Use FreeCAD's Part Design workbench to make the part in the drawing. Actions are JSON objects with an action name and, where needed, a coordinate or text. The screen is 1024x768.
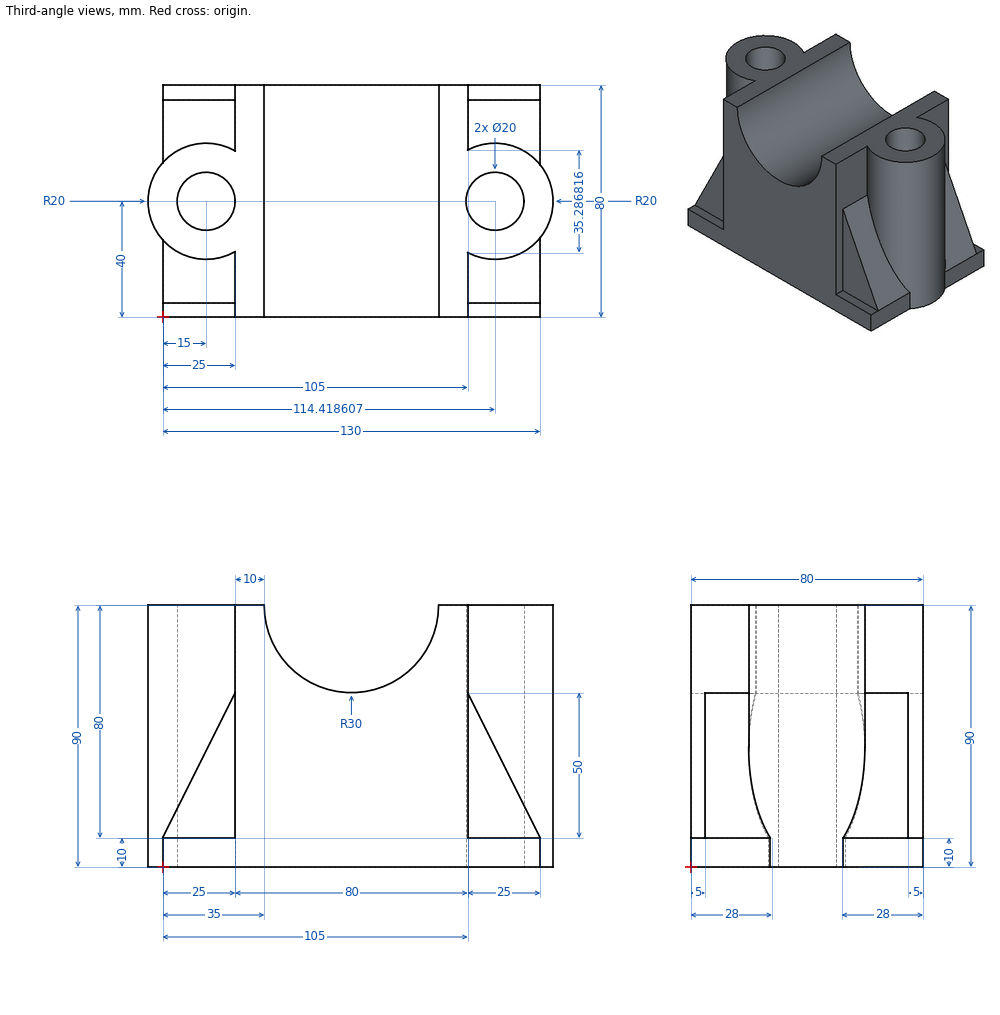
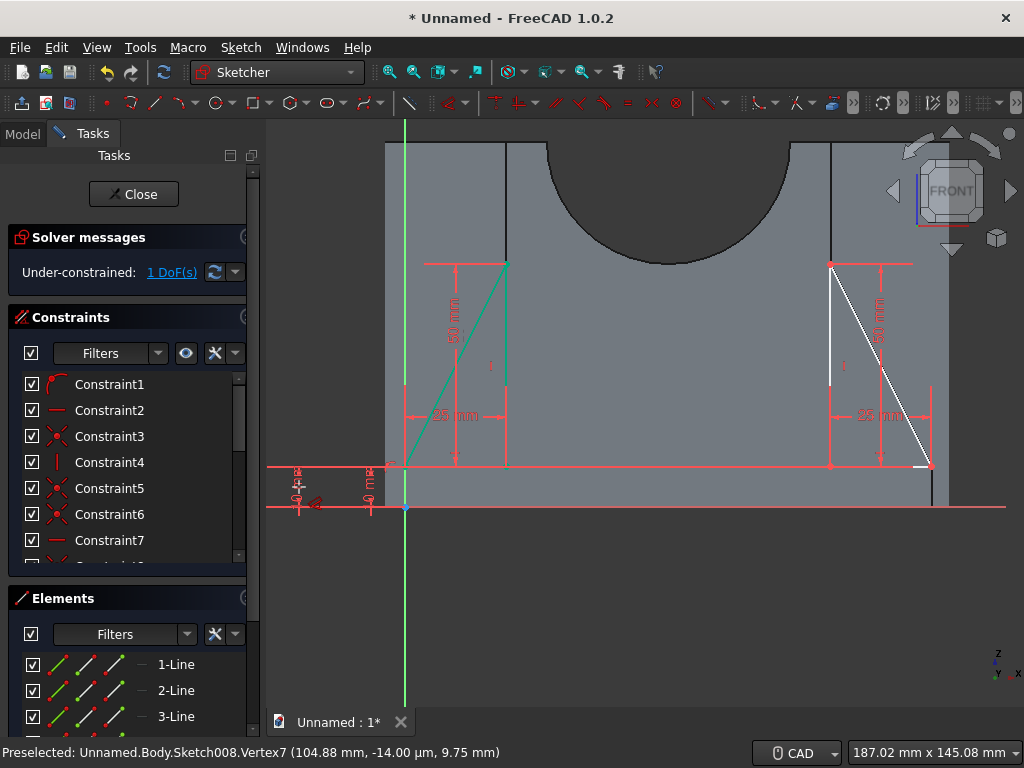
{"action": "left_click", "coordinate": [830, 467]}
{"action": "left_click", "coordinate": [618, 541]}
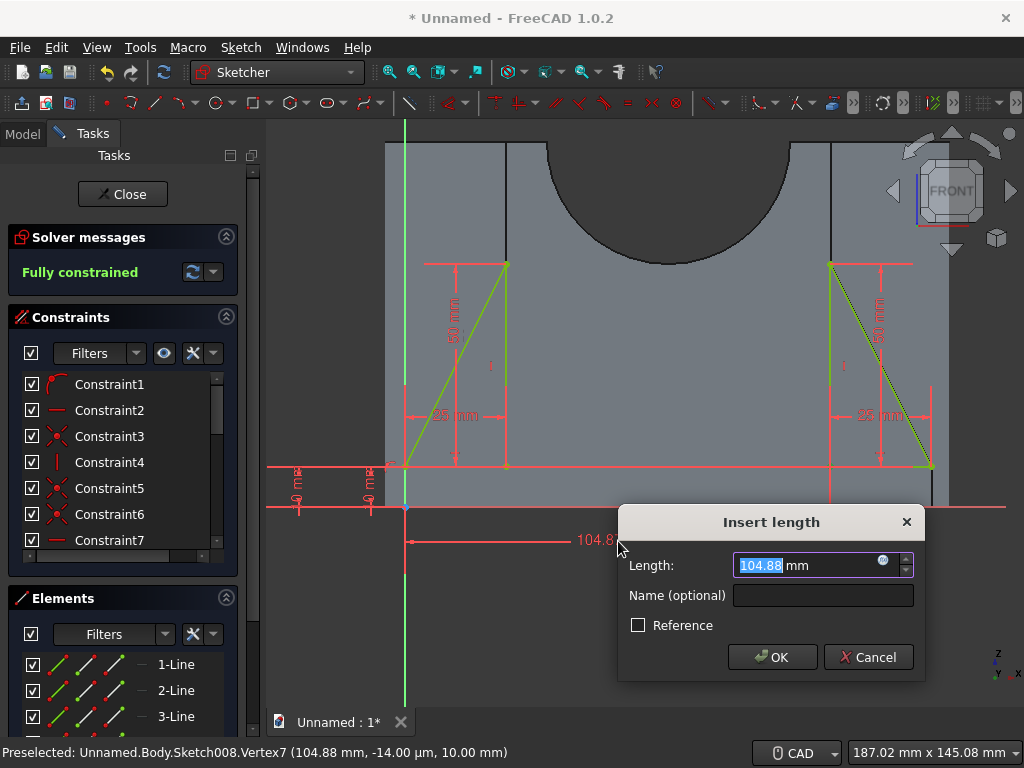
{"action": "type", "text": "105"}
{"action": "key", "text": "Return"}
{"action": "key", "text": "Escape"}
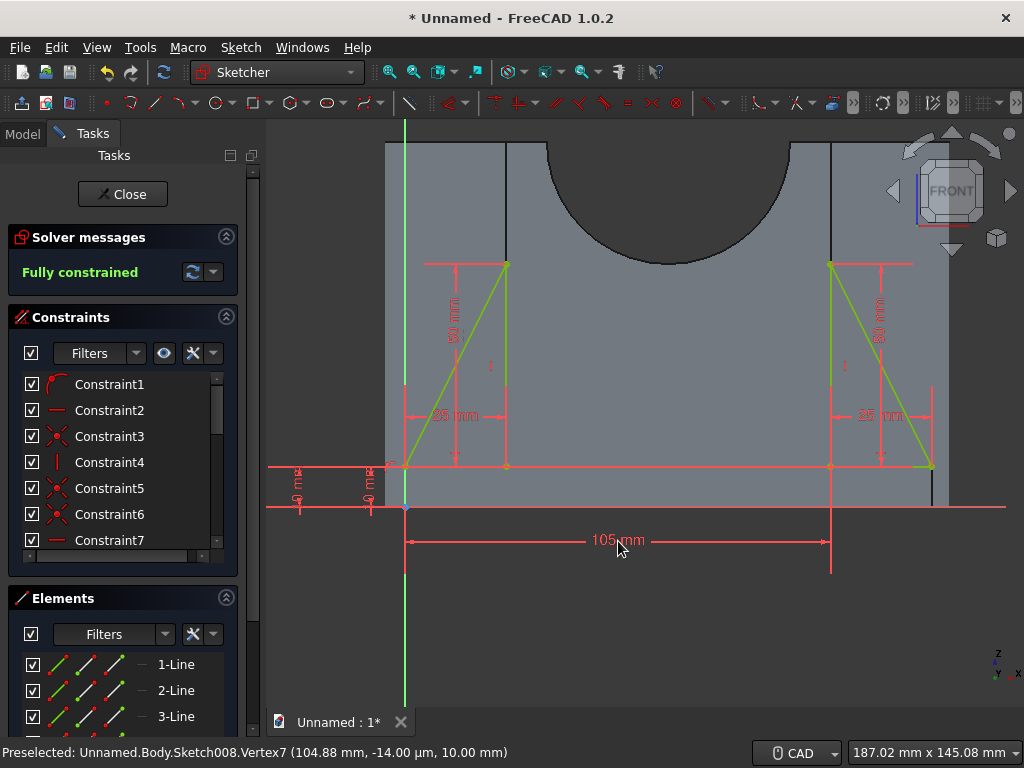
{"action": "left_click", "coordinate": [123, 194]}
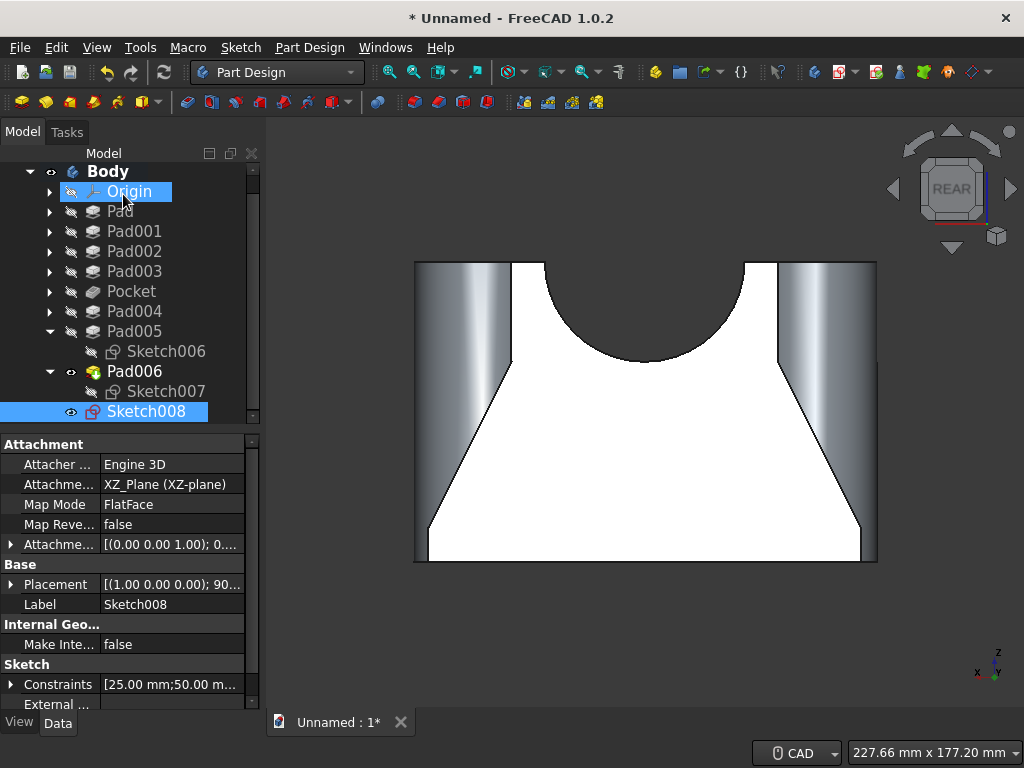
{"action": "left_click", "coordinate": [188, 102]}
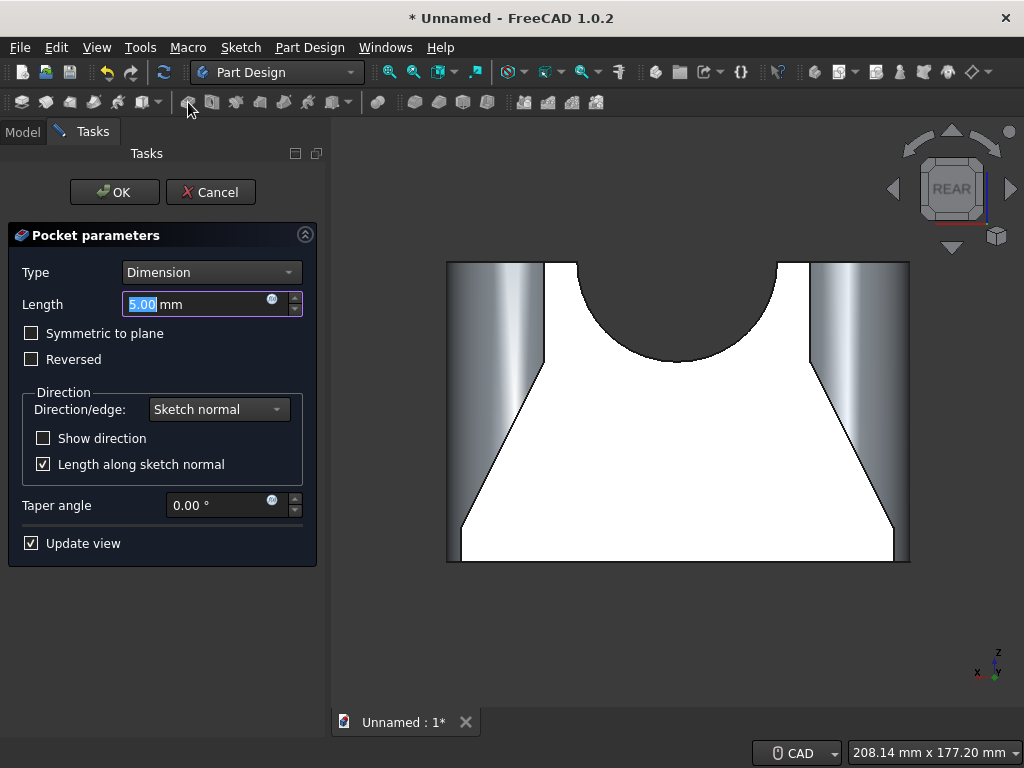
{"action": "type", "text": "5"}
{"action": "key", "text": "Tab"}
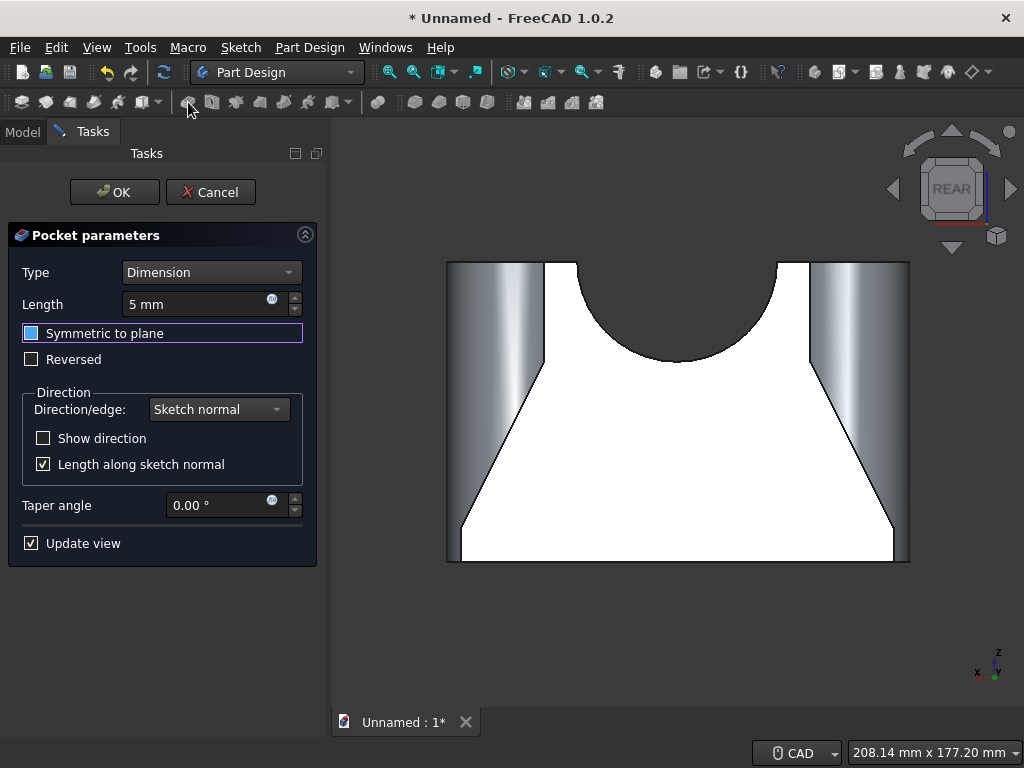
{"action": "left_click", "coordinate": [115, 192]}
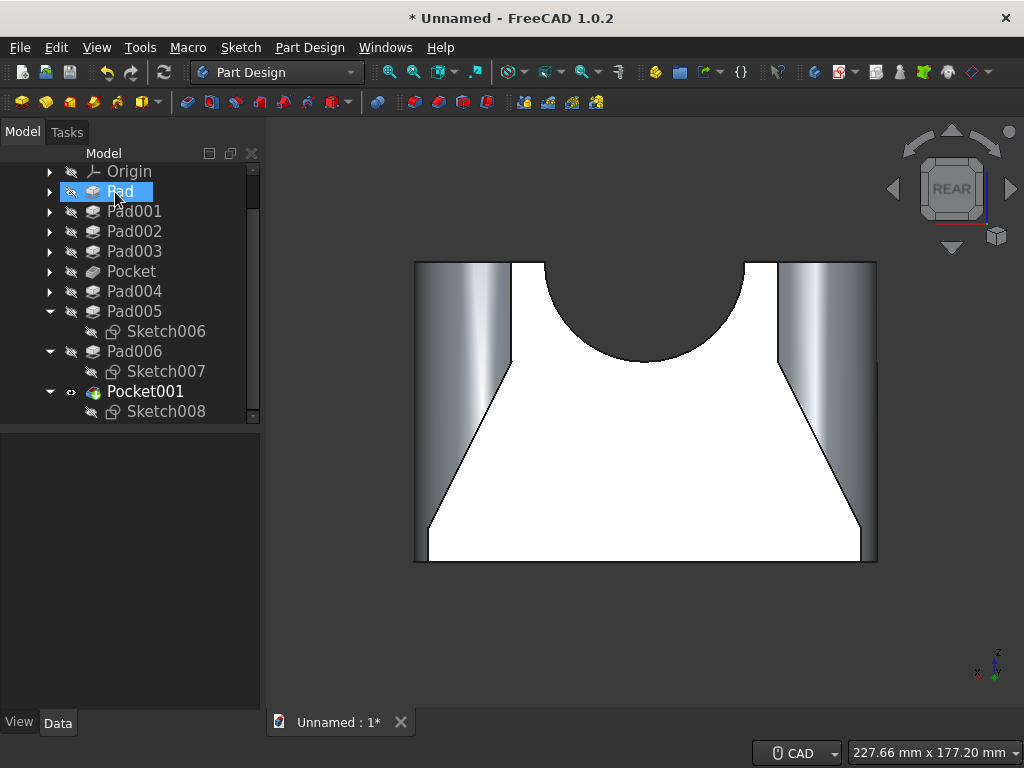
{"action": "left_click", "coordinate": [706, 454]}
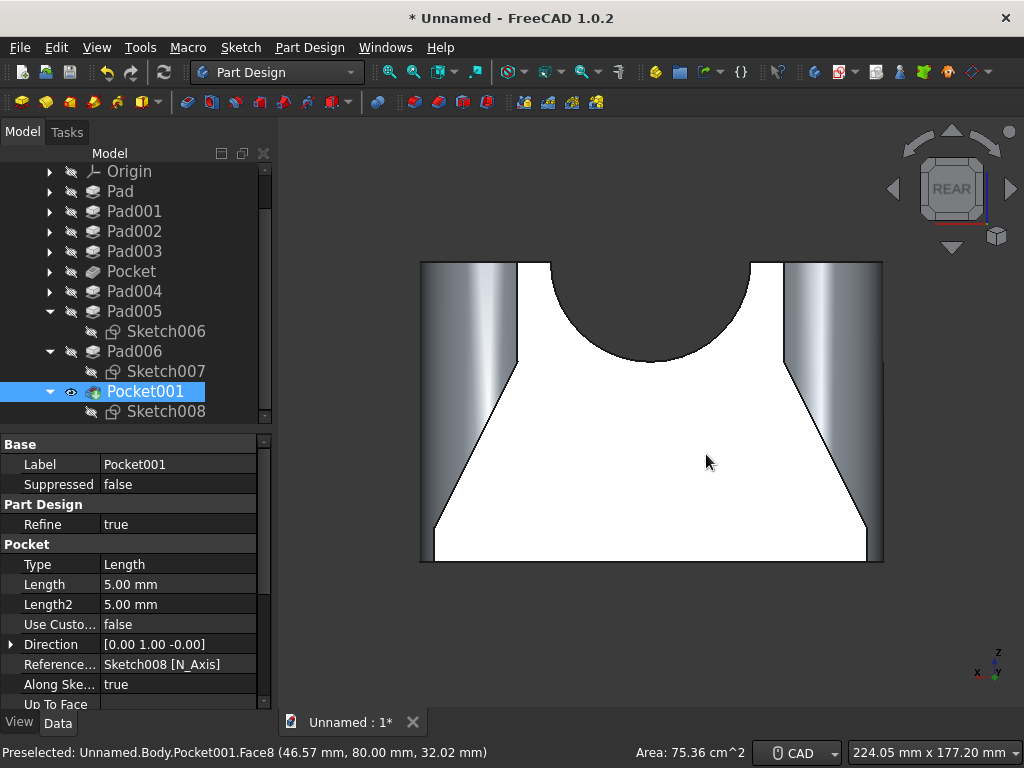
{"action": "left_click", "coordinate": [840, 72]}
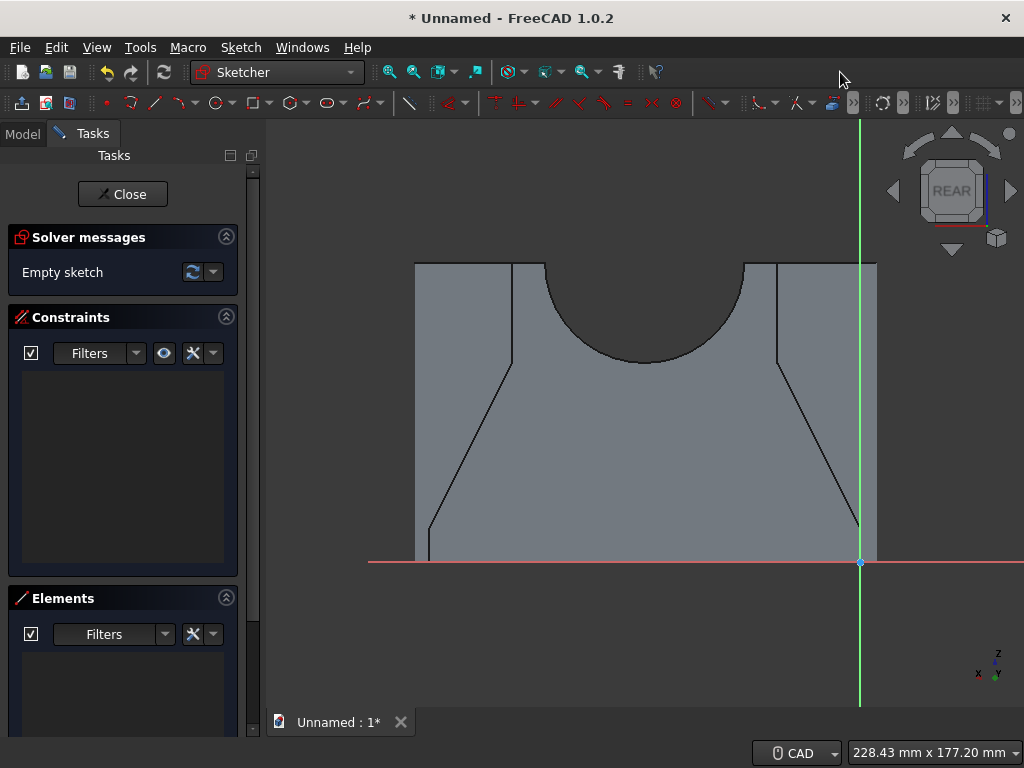
{"action": "scroll", "coordinate": [294, 189], "scroll_direction": "down", "scroll_amount": 1}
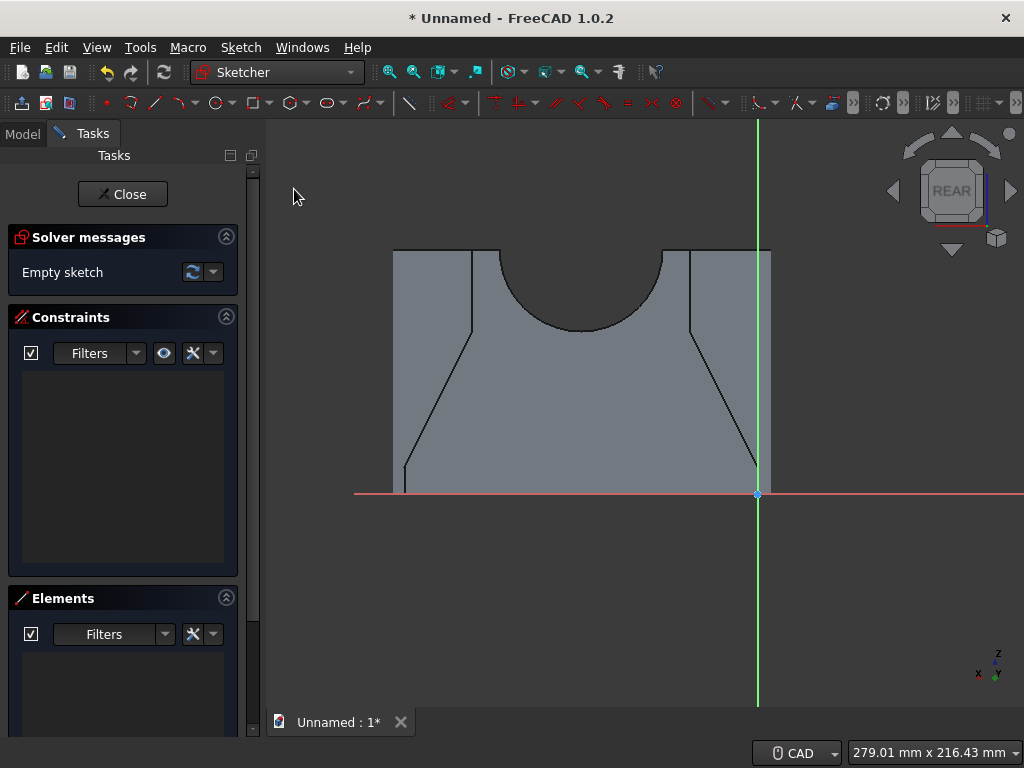
{"action": "left_click", "coordinate": [132, 104]}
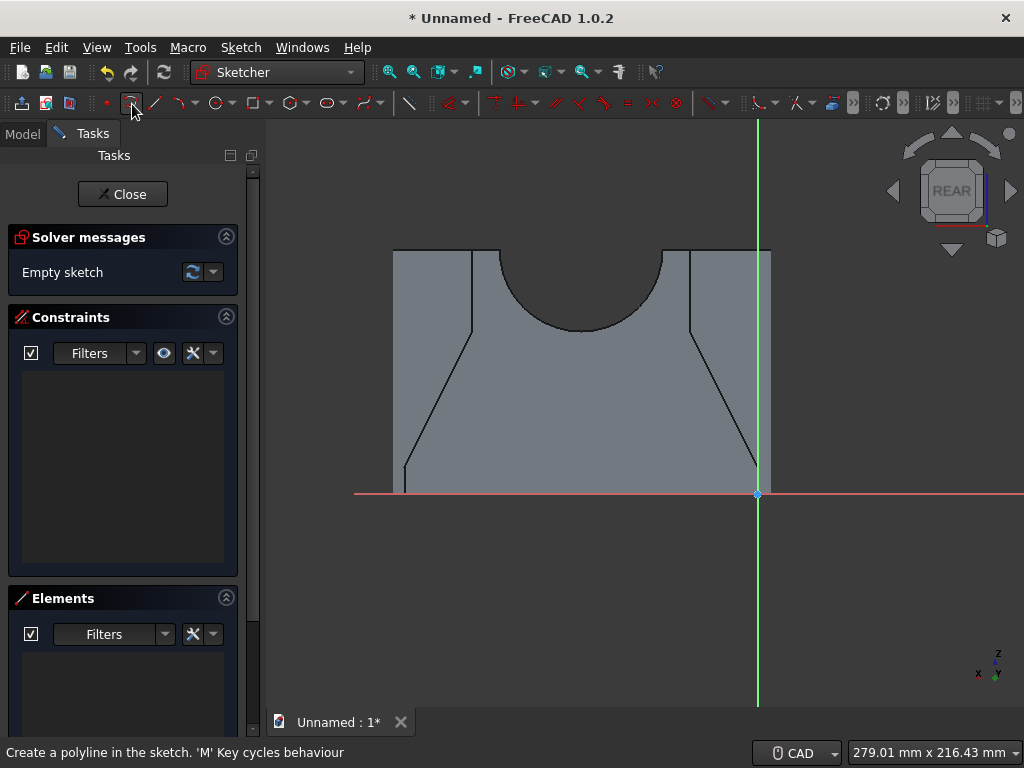
{"action": "left_click", "coordinate": [758, 467]}
{"action": "left_click", "coordinate": [690, 331]}
{"action": "left_click", "coordinate": [690, 467]}
{"action": "left_click", "coordinate": [758, 468]}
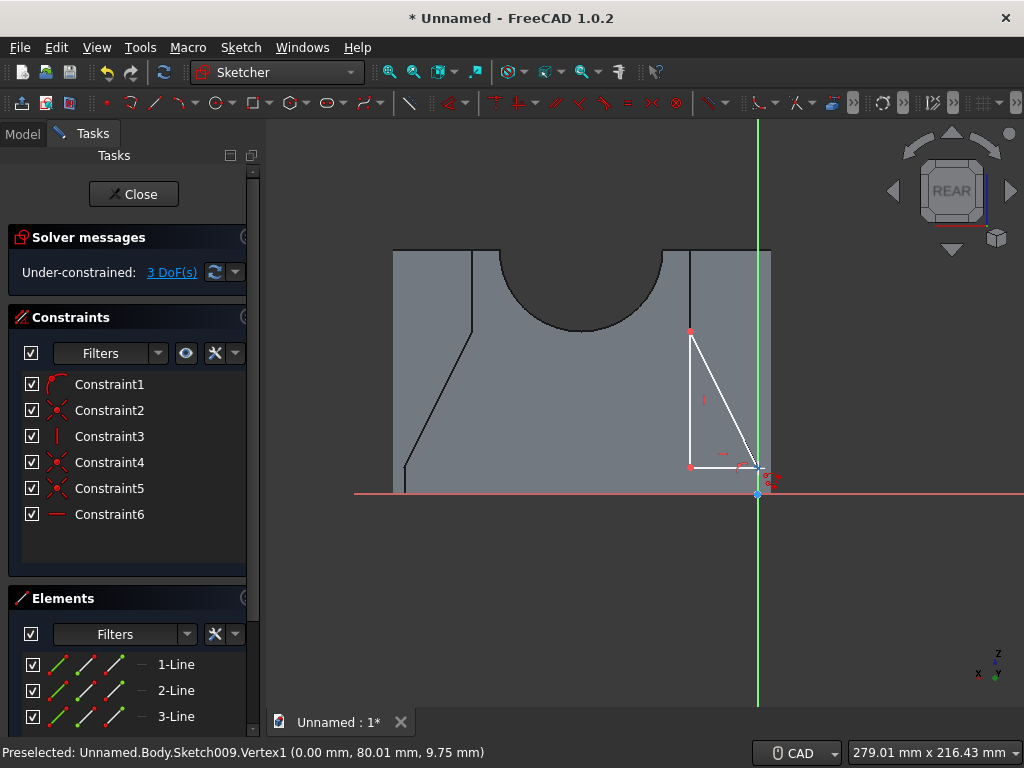
{"action": "left_click", "coordinate": [472, 467]}
{"action": "left_click", "coordinate": [472, 331]}
{"action": "left_click", "coordinate": [405, 467]}
{"action": "left_click", "coordinate": [472, 468]}
{"action": "key", "text": "Escape"}
{"action": "key", "text": "Escape"}